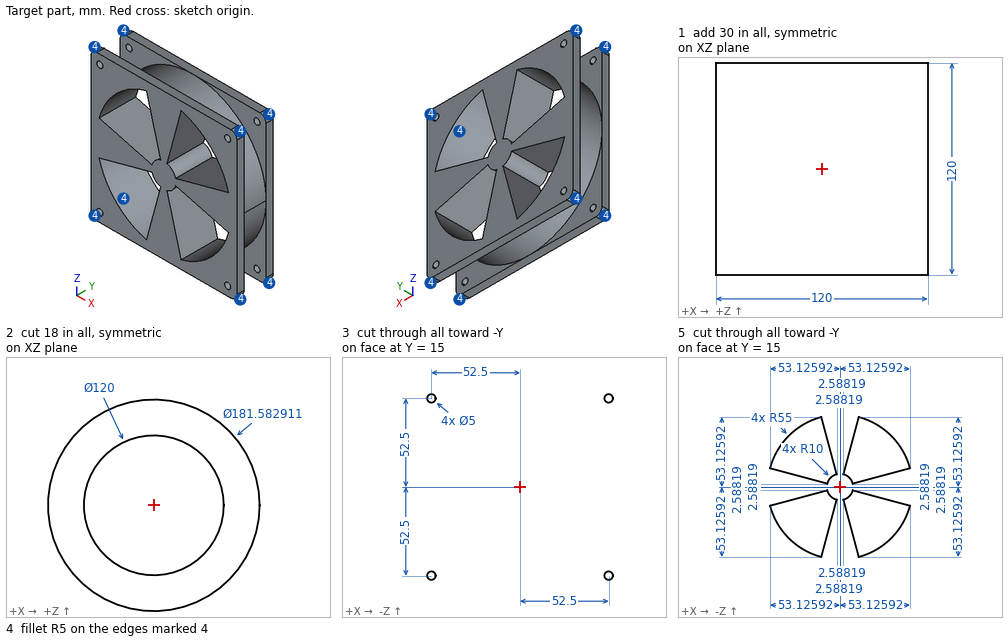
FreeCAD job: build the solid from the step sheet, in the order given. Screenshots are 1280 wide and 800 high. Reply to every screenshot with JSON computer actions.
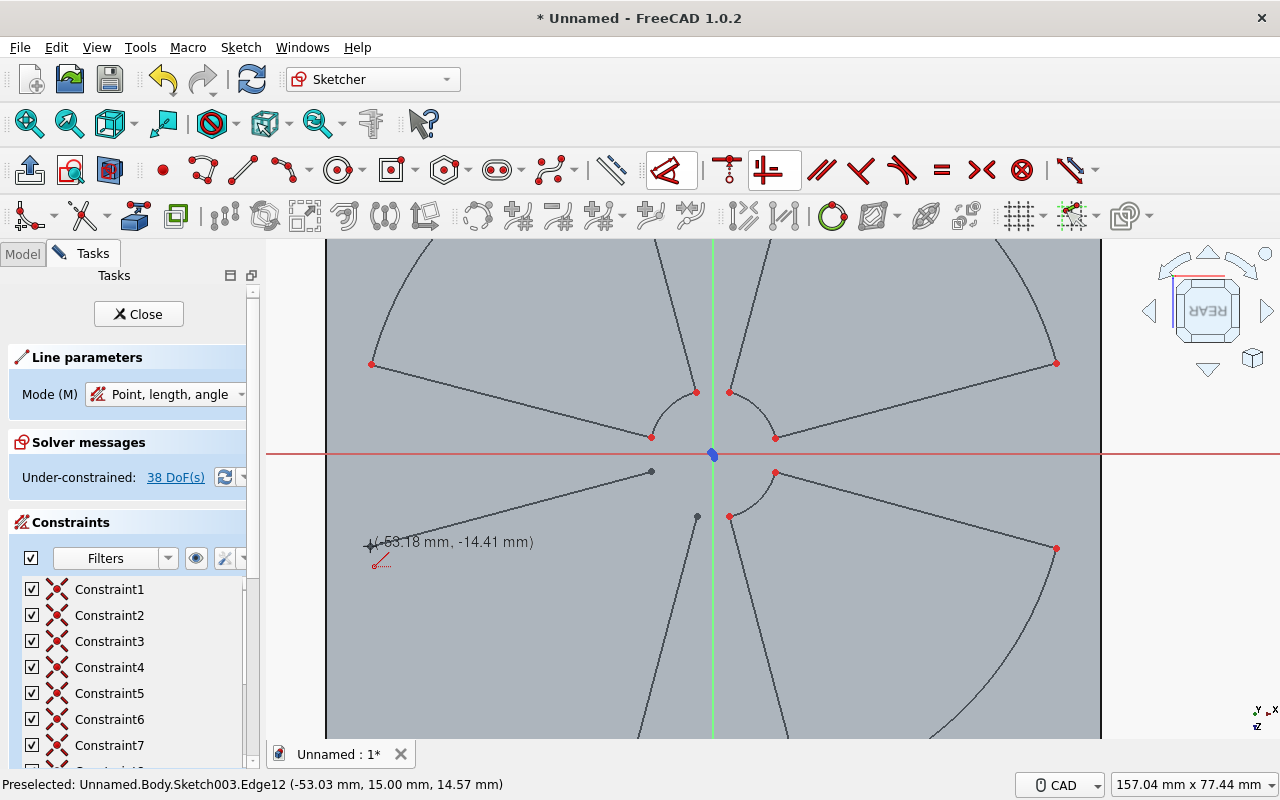
{"action": "left_click", "coordinate": [284, 170]}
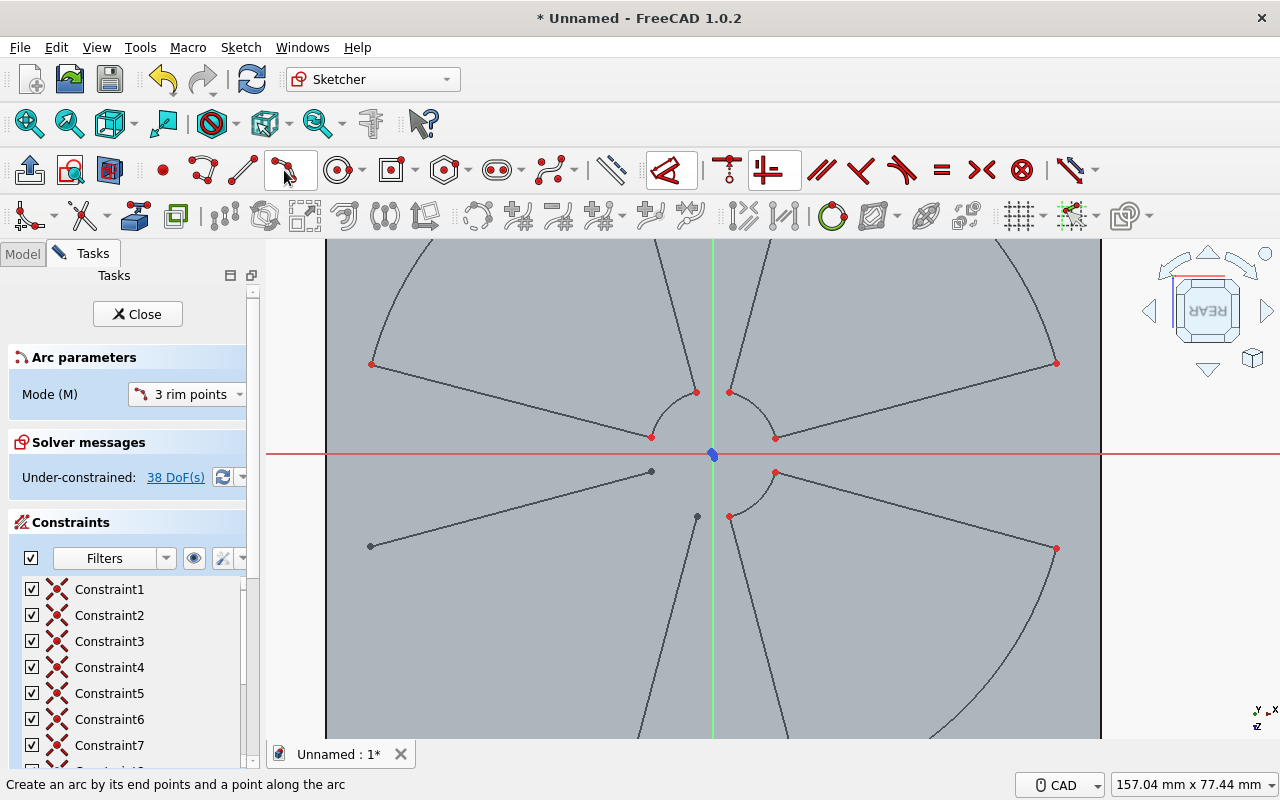
{"action": "left_click", "coordinate": [697, 517]}
{"action": "left_click", "coordinate": [651, 472]}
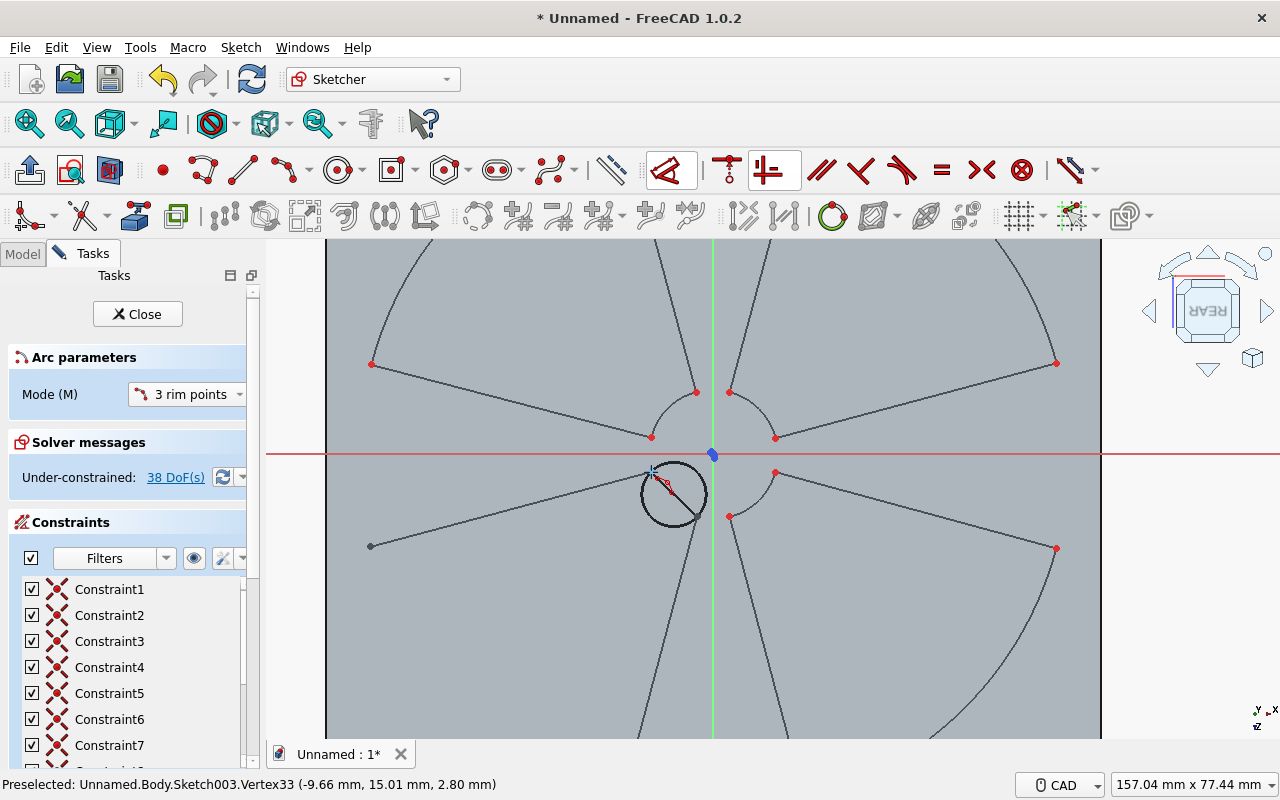
{"action": "scroll", "coordinate": [668, 500], "scroll_direction": "up", "scroll_amount": 4}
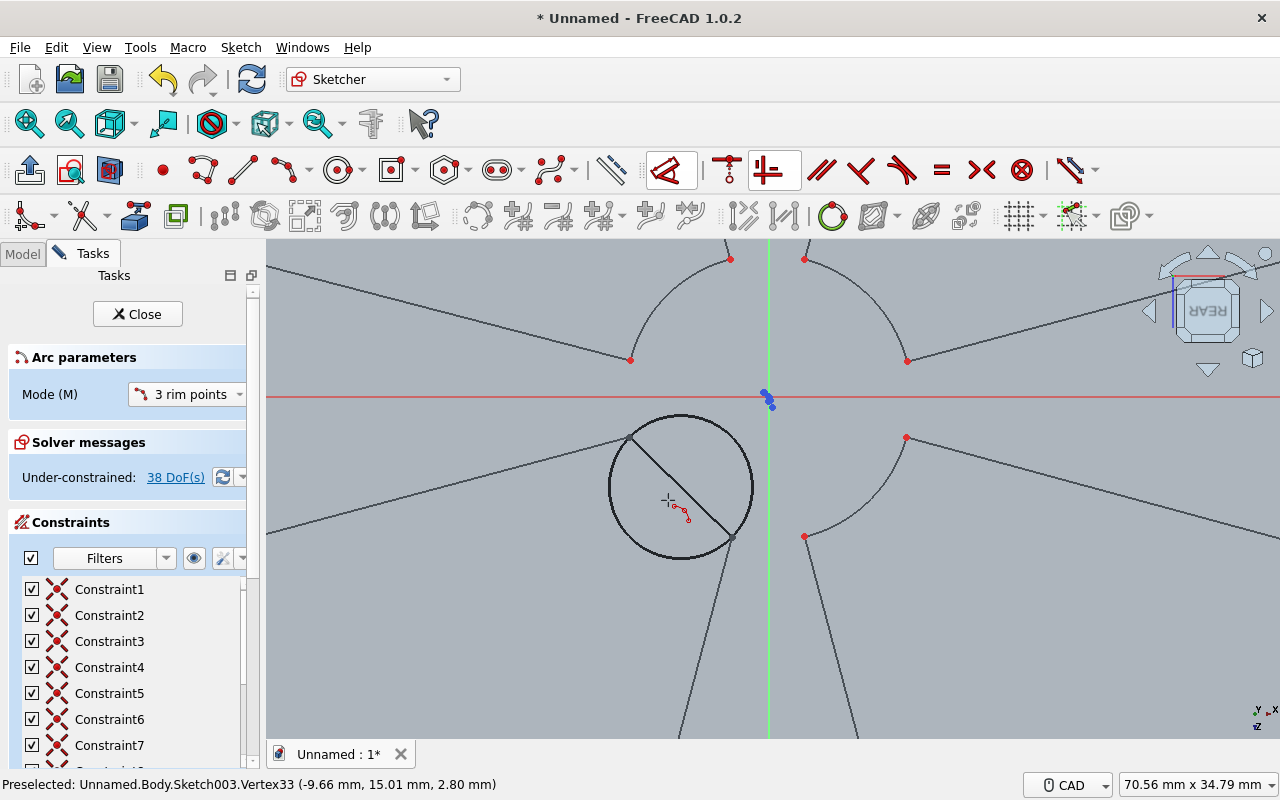
{"action": "left_click", "coordinate": [667, 498]}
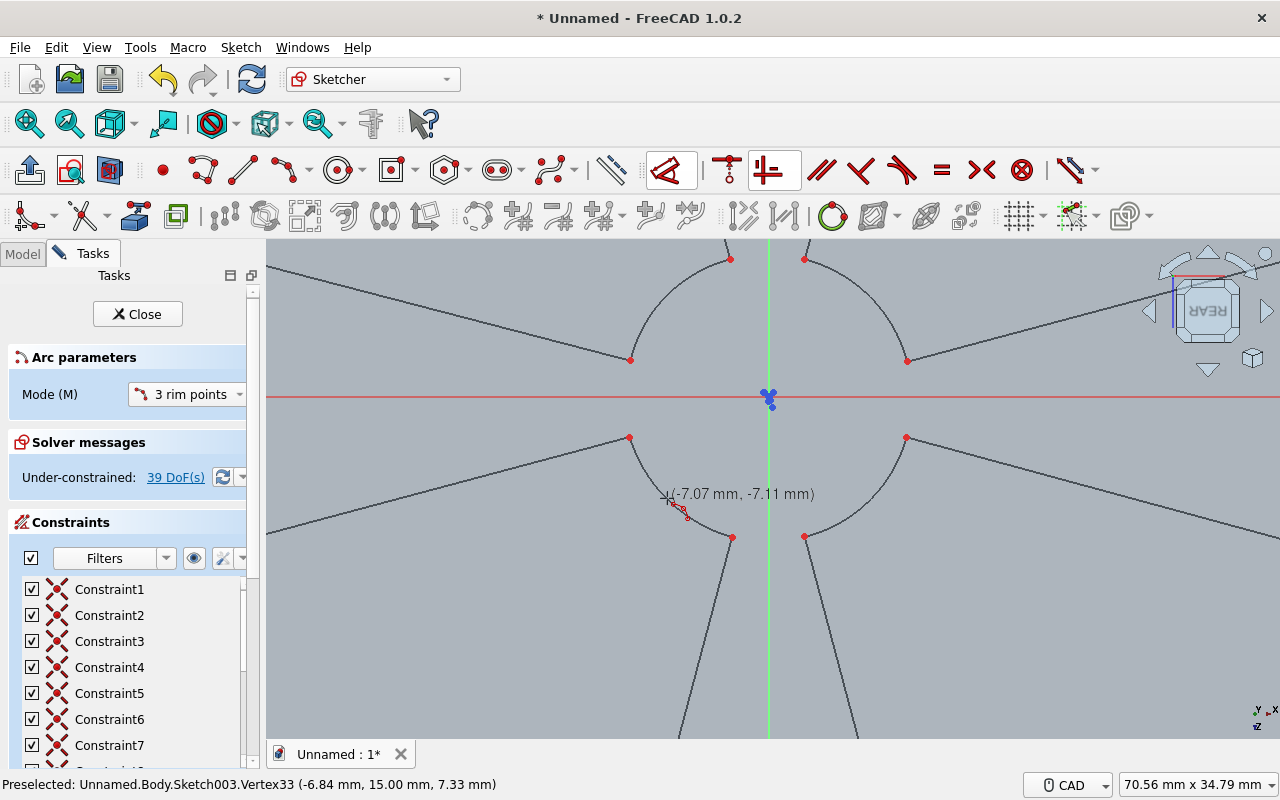
{"action": "scroll", "coordinate": [688, 512], "scroll_direction": "down", "scroll_amount": 8}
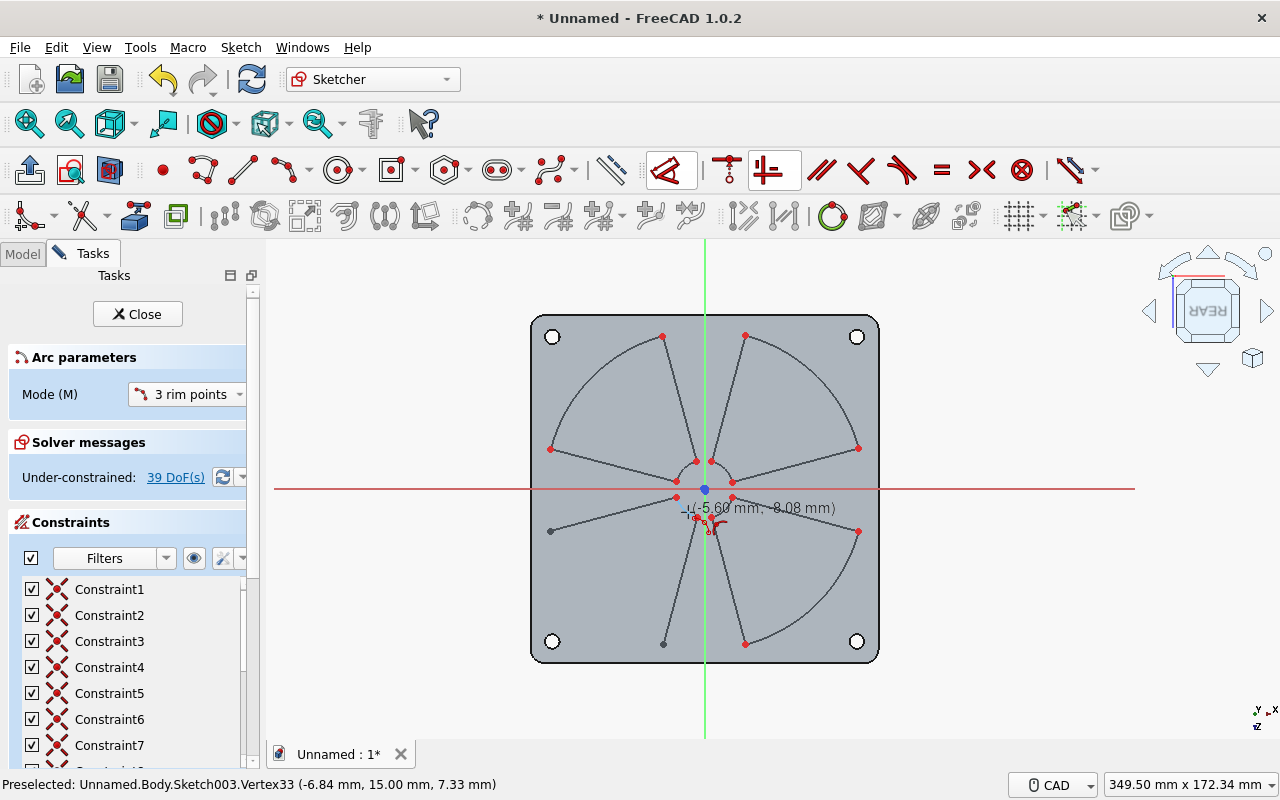
{"action": "left_click", "coordinate": [550, 531]}
{"action": "left_click", "coordinate": [663, 645]}
{"action": "left_click", "coordinate": [592, 602]}
{"action": "key", "text": "Escape"}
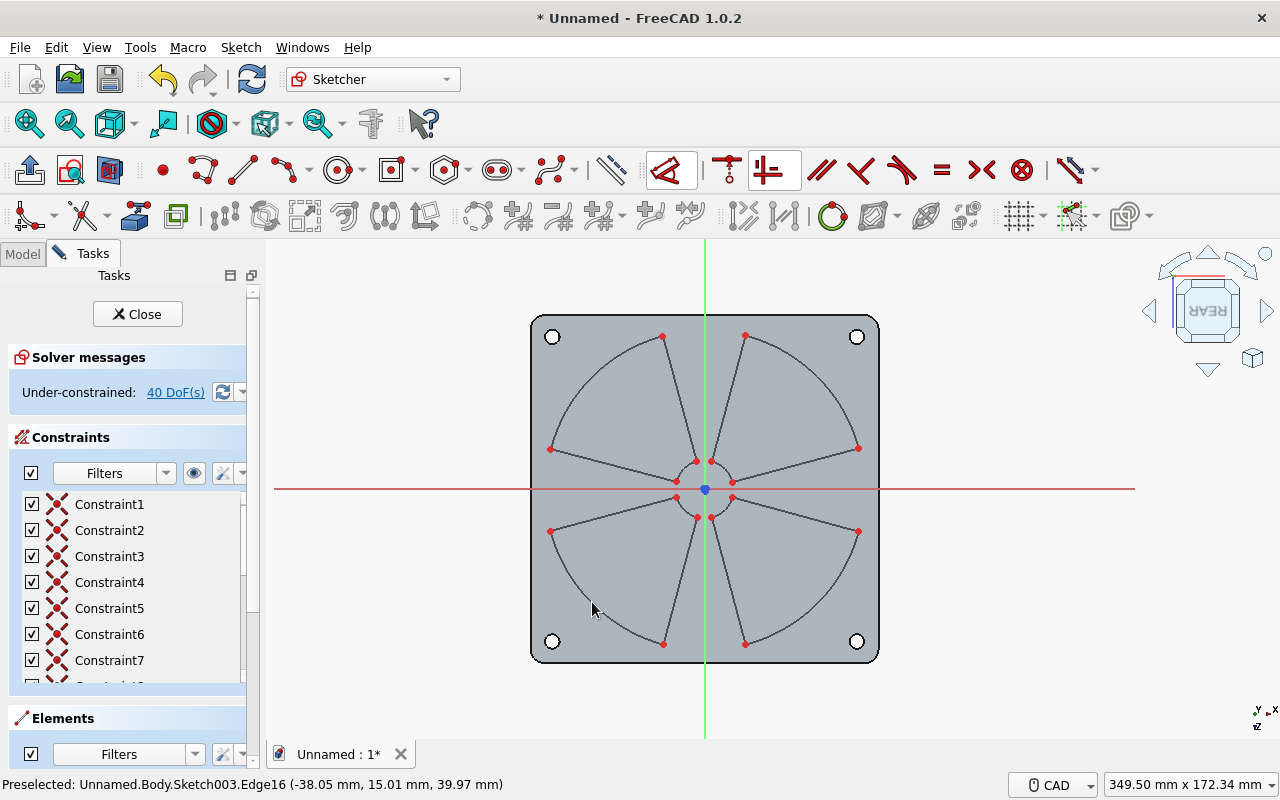
{"action": "left_click", "coordinate": [617, 356]}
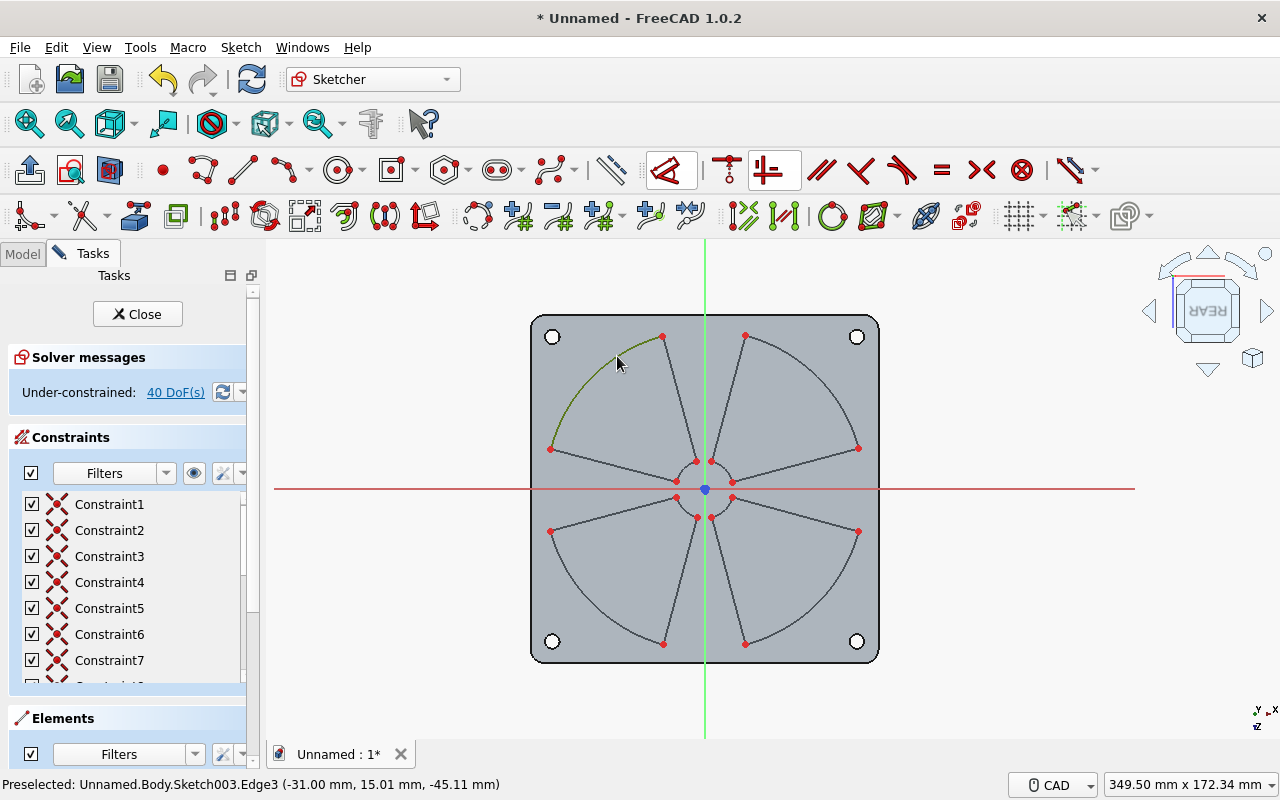
{"action": "scroll", "coordinate": [689, 465], "scroll_direction": "up", "scroll_amount": 3}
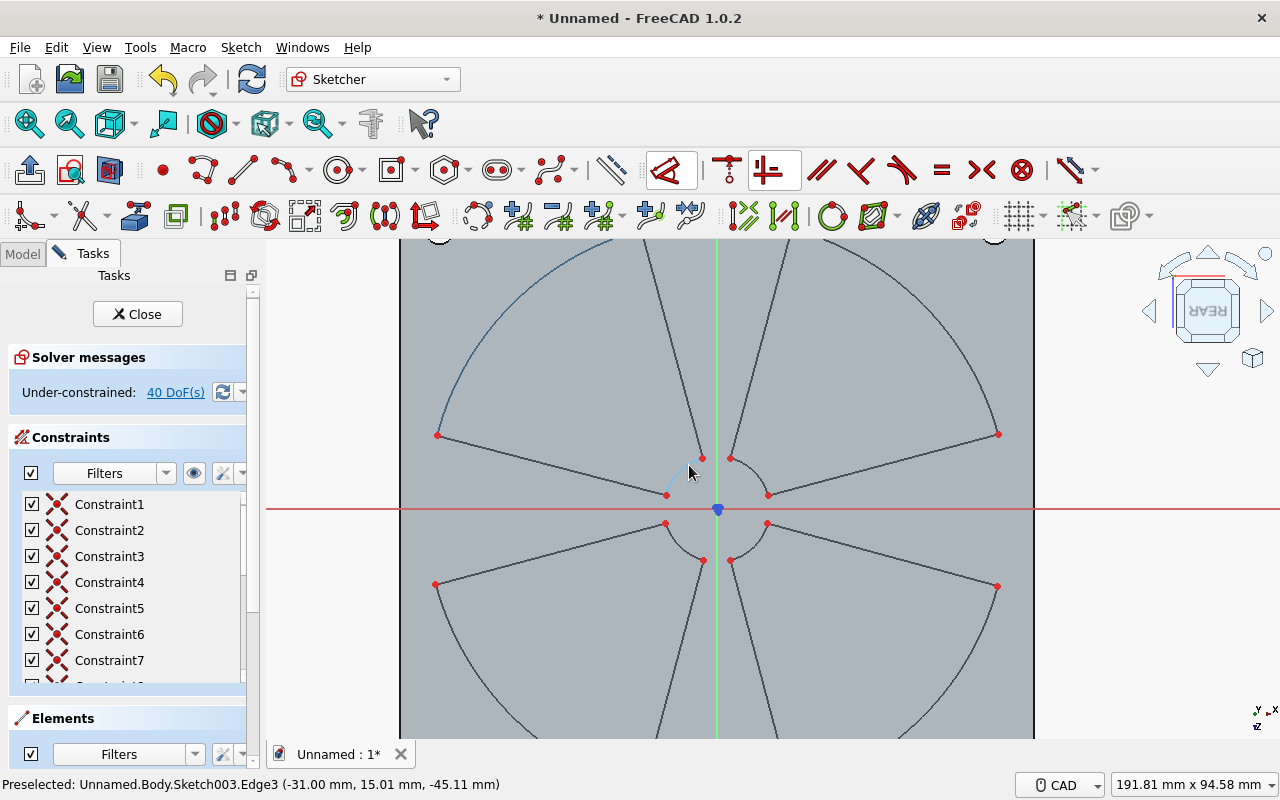
{"action": "left_click", "coordinate": [688, 465]}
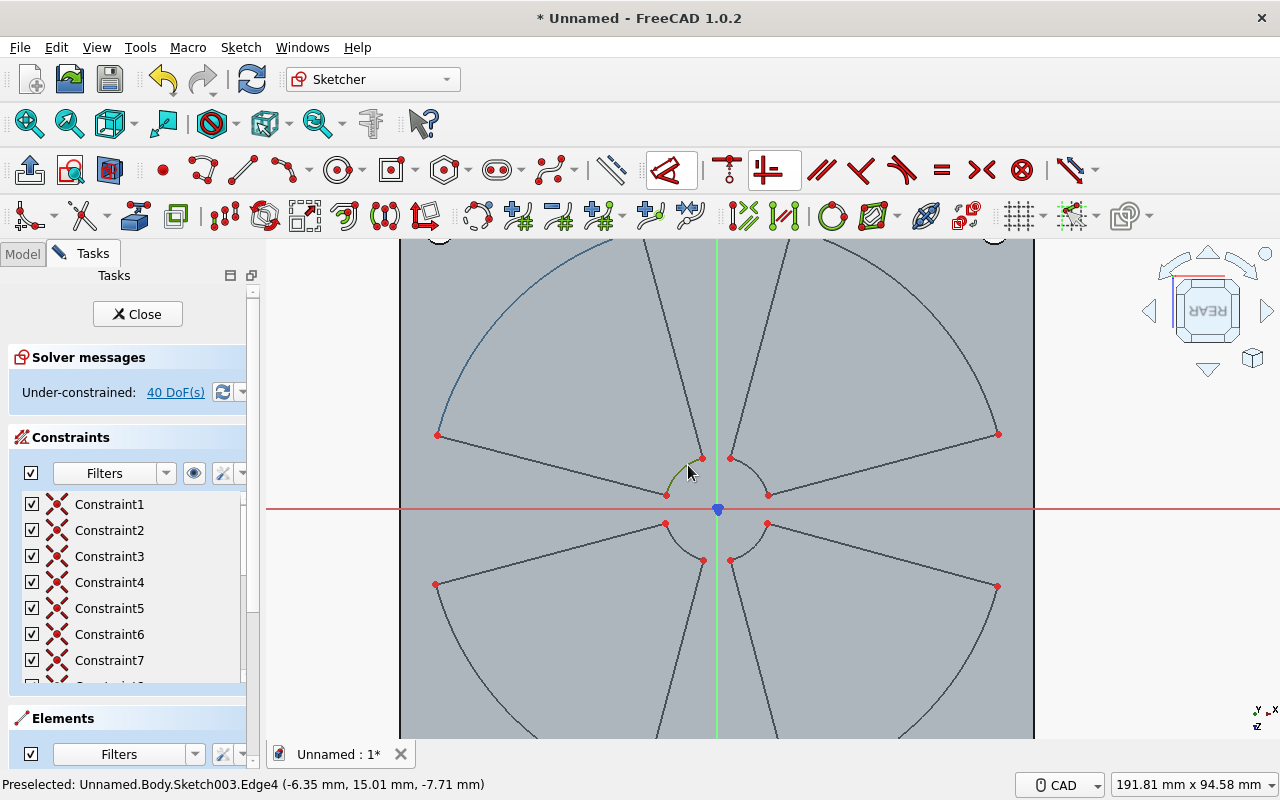
{"action": "left_click", "coordinate": [728, 170]}